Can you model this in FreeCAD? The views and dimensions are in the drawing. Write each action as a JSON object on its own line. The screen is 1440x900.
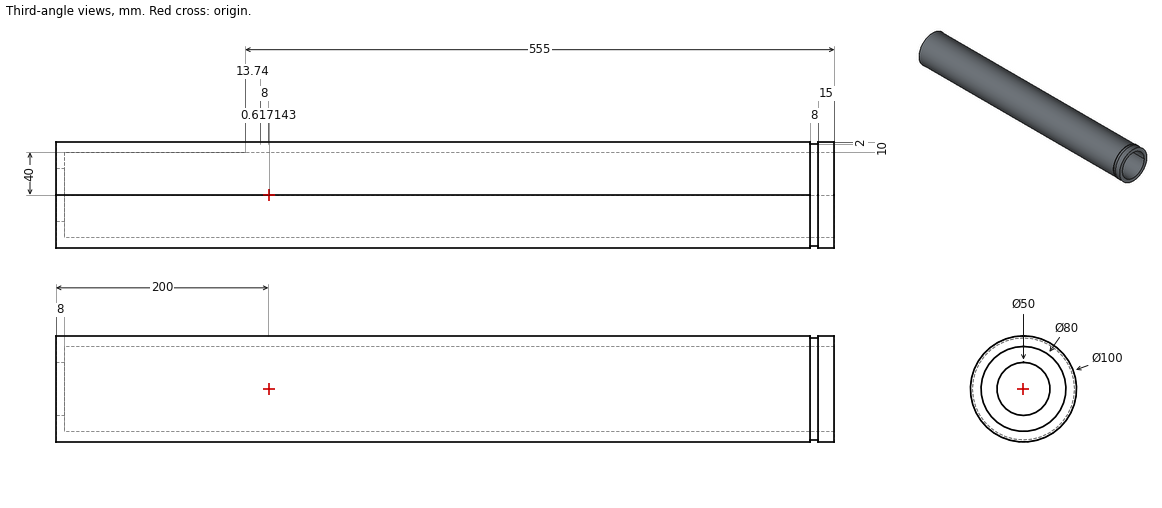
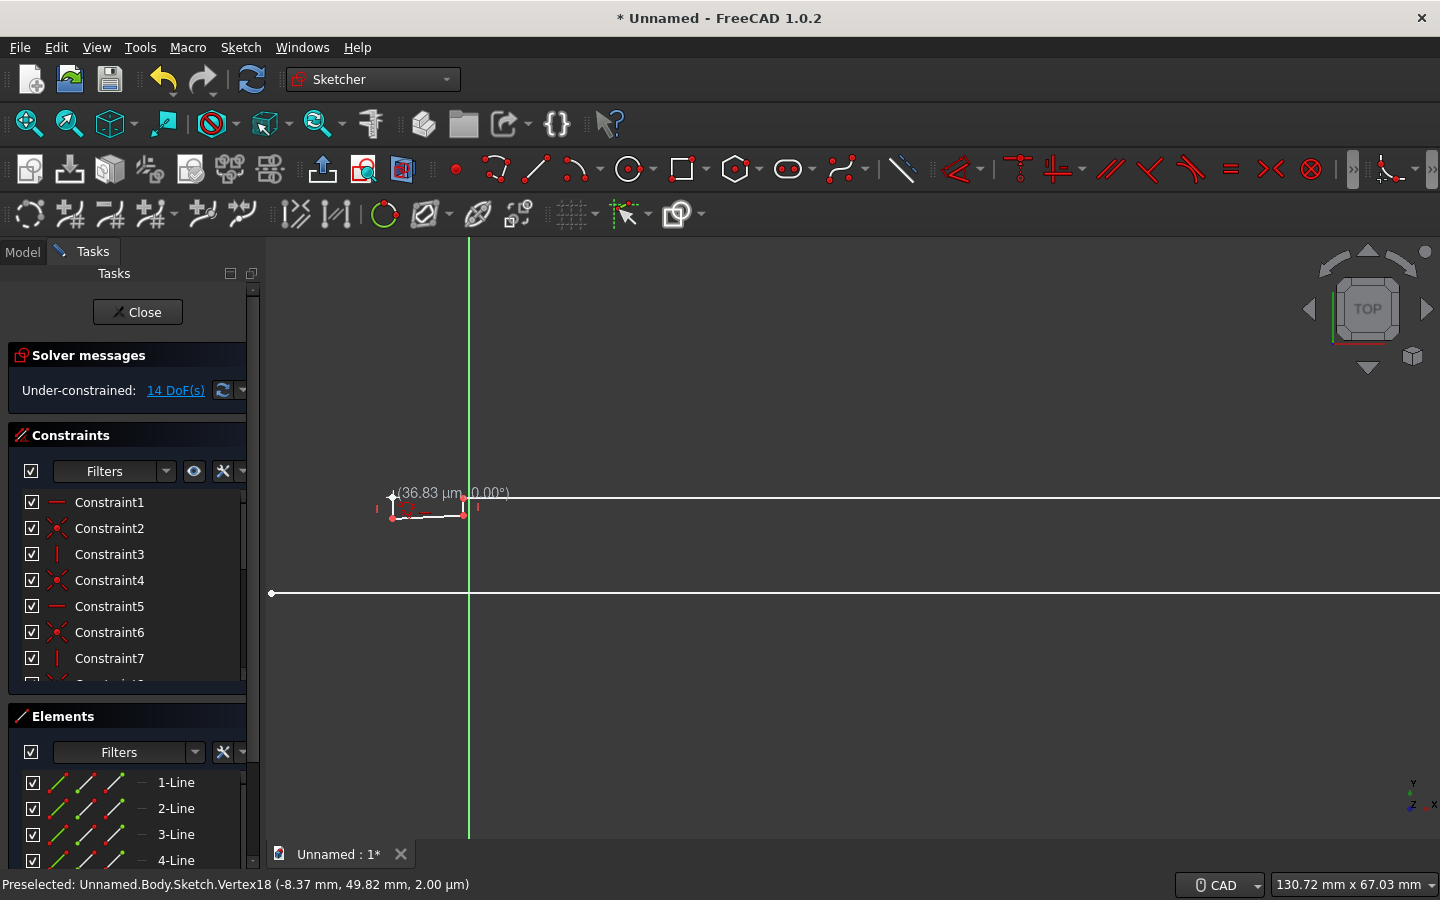
{"action": "scroll", "coordinate": [475, 509], "scroll_direction": "down", "scroll_amount": 10}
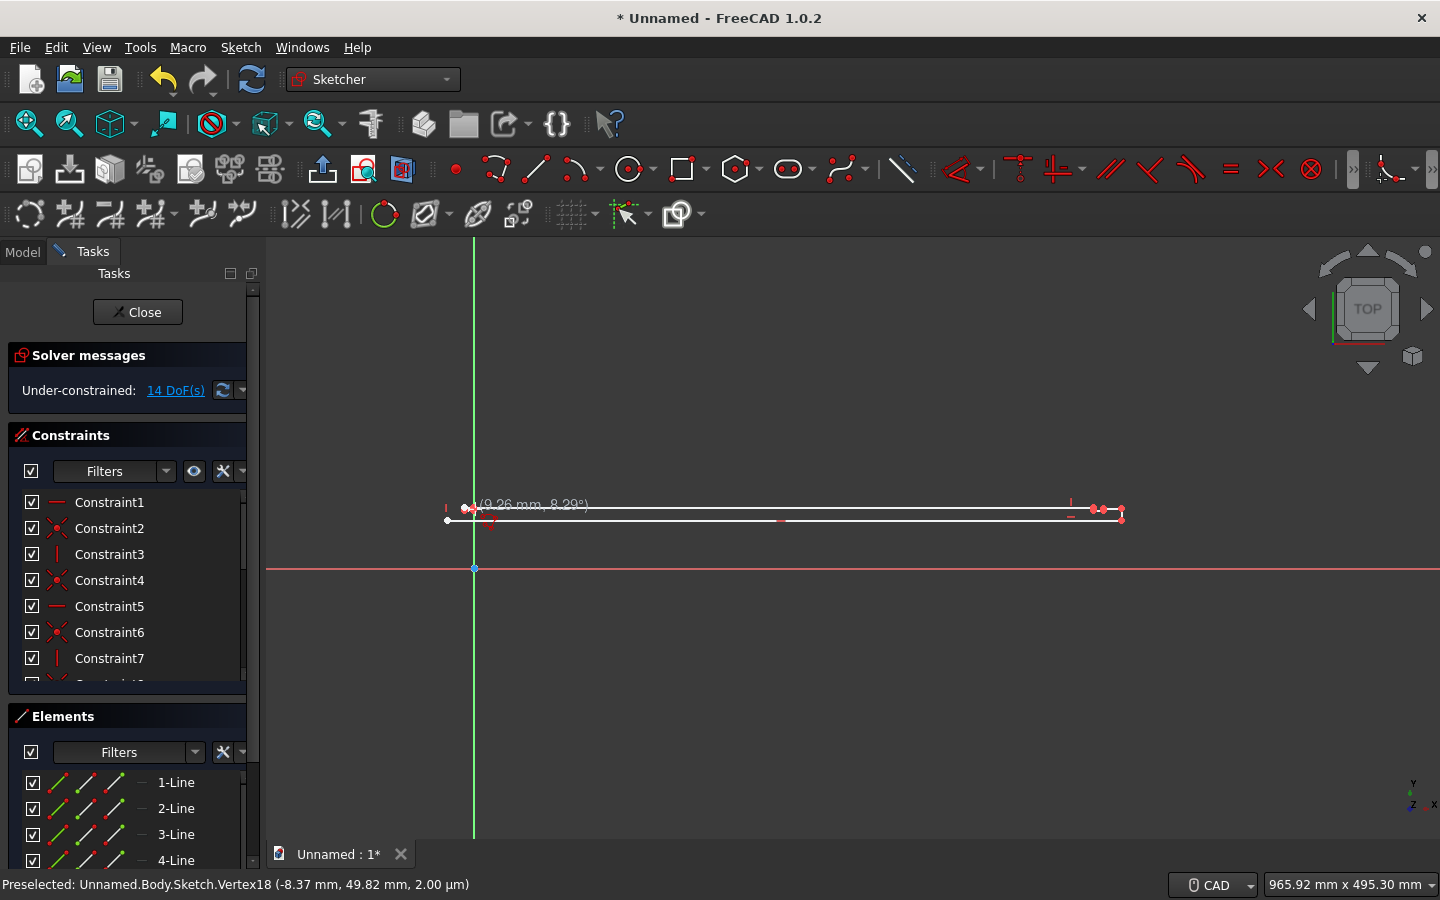
{"action": "scroll", "coordinate": [447, 508], "scroll_direction": "up", "scroll_amount": 2}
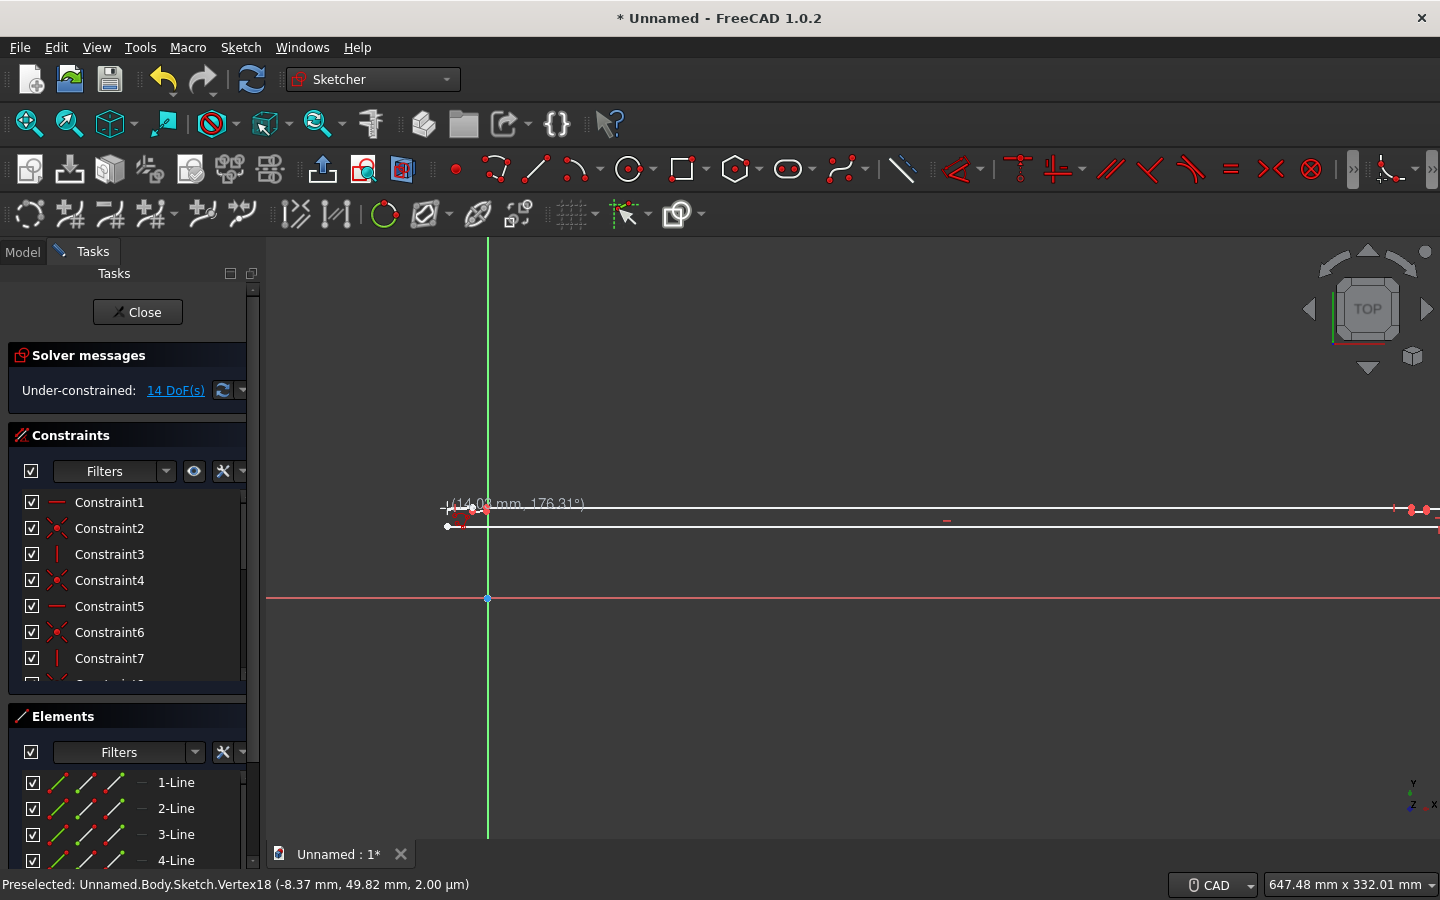
{"action": "left_click", "coordinate": [447, 507]}
{"action": "left_click", "coordinate": [448, 527]}
{"action": "key", "text": "Escape"}
{"action": "key", "text": "Escape"}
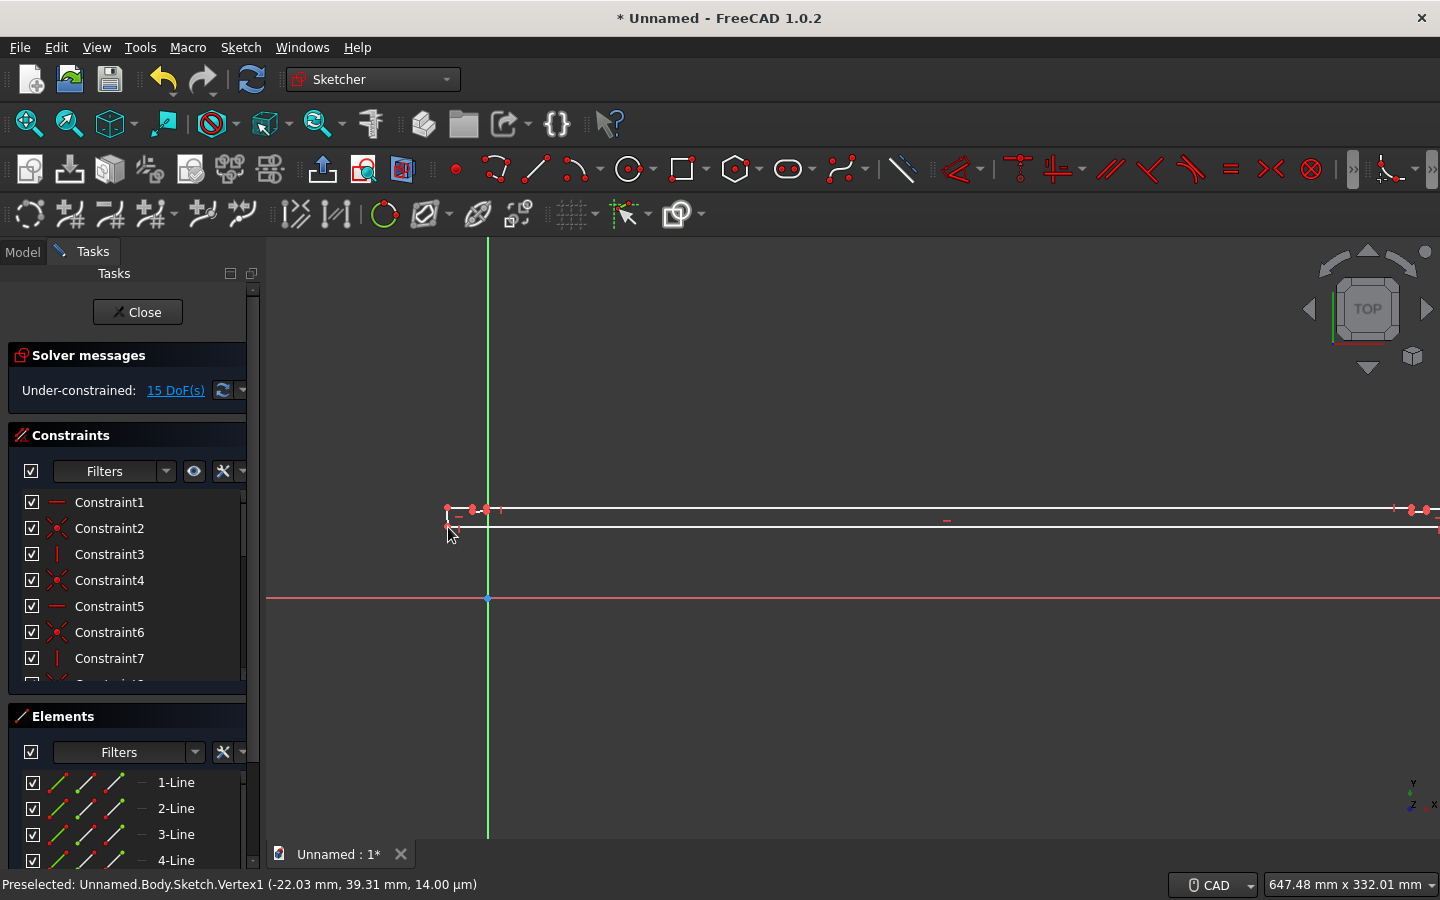
{"action": "scroll", "coordinate": [447, 508], "scroll_direction": "down", "scroll_amount": 2}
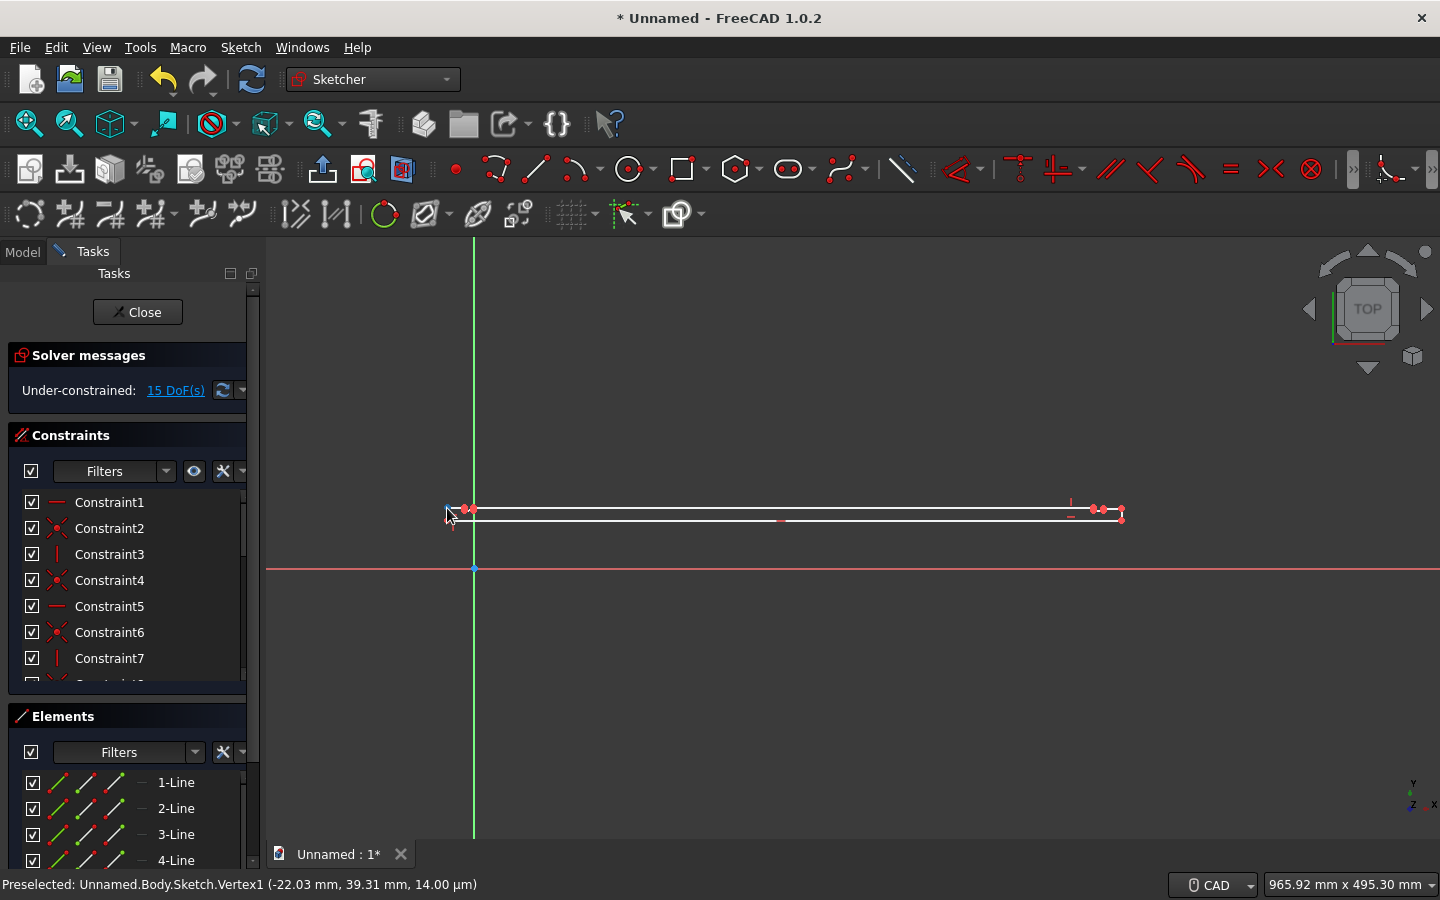
{"action": "scroll", "coordinate": [1099, 511], "scroll_direction": "up", "scroll_amount": 6}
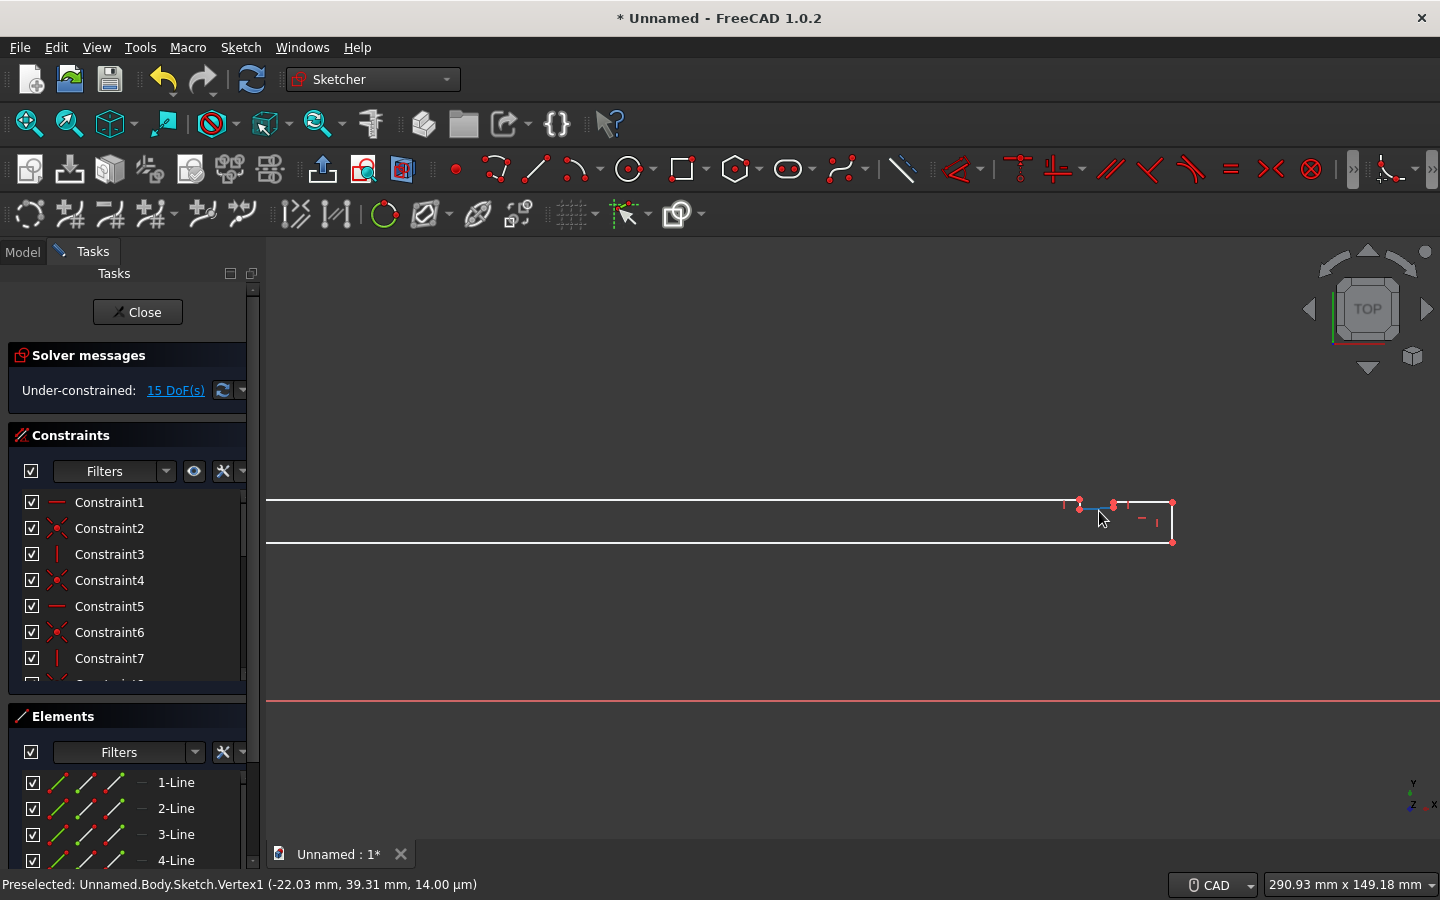
{"action": "left_click", "coordinate": [1096, 509]}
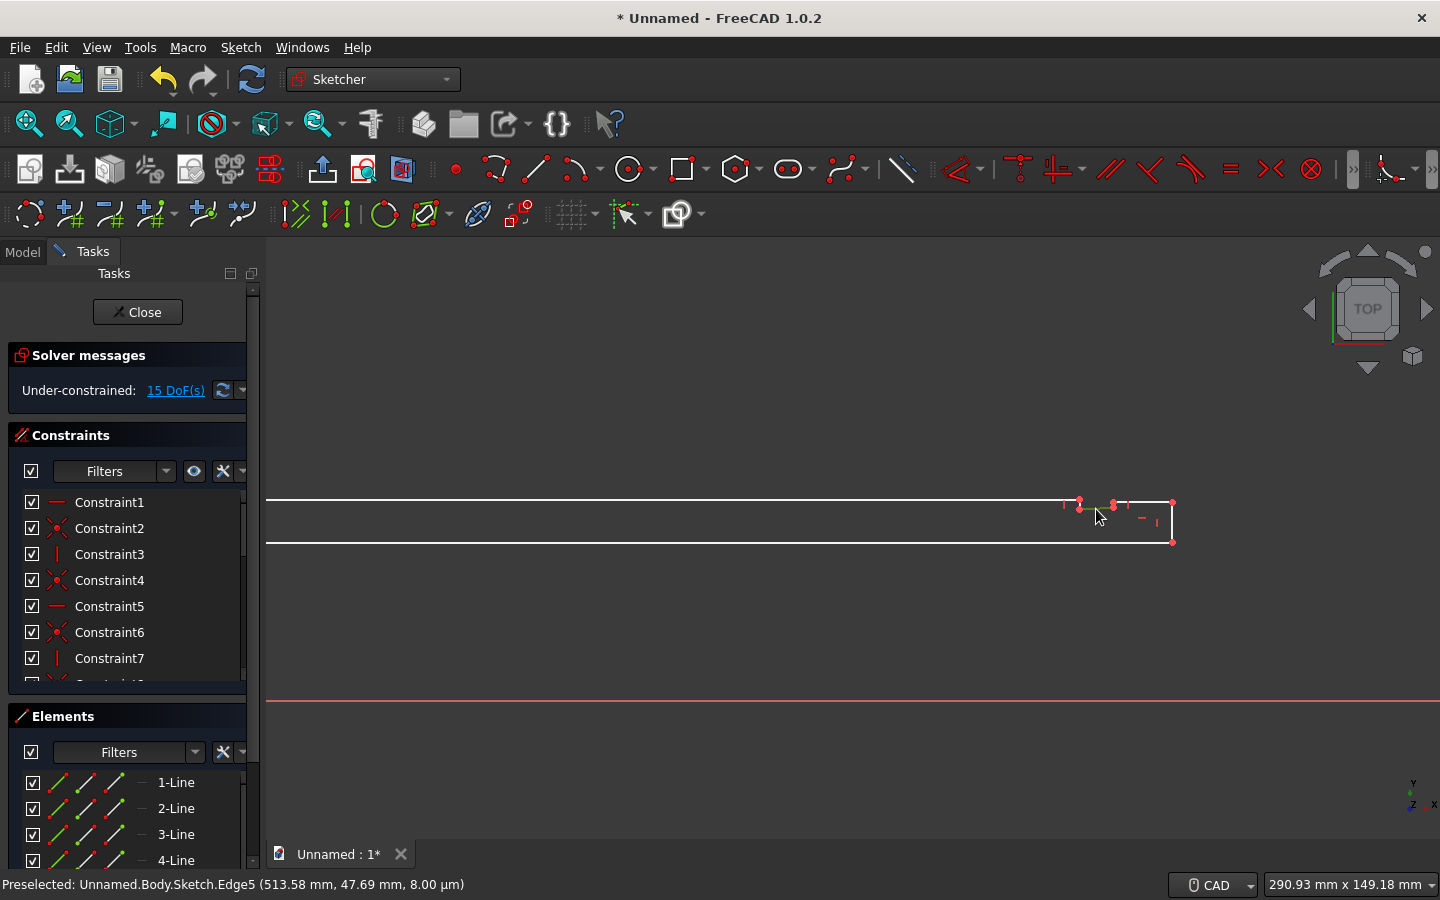
{"action": "key", "text": "h"}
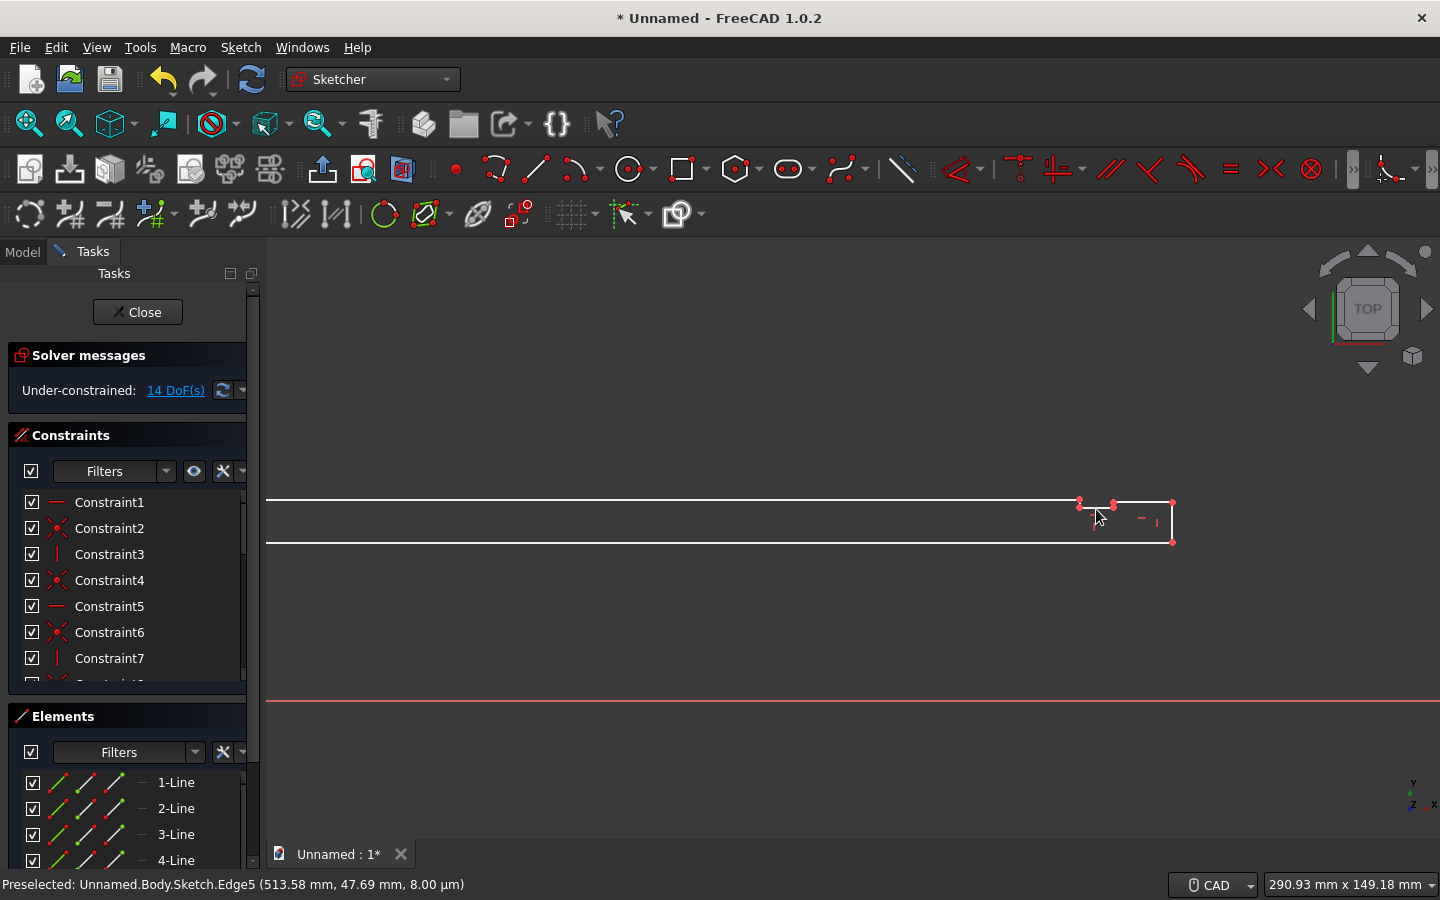
{"action": "scroll", "coordinate": [1100, 511], "scroll_direction": "down", "scroll_amount": 6}